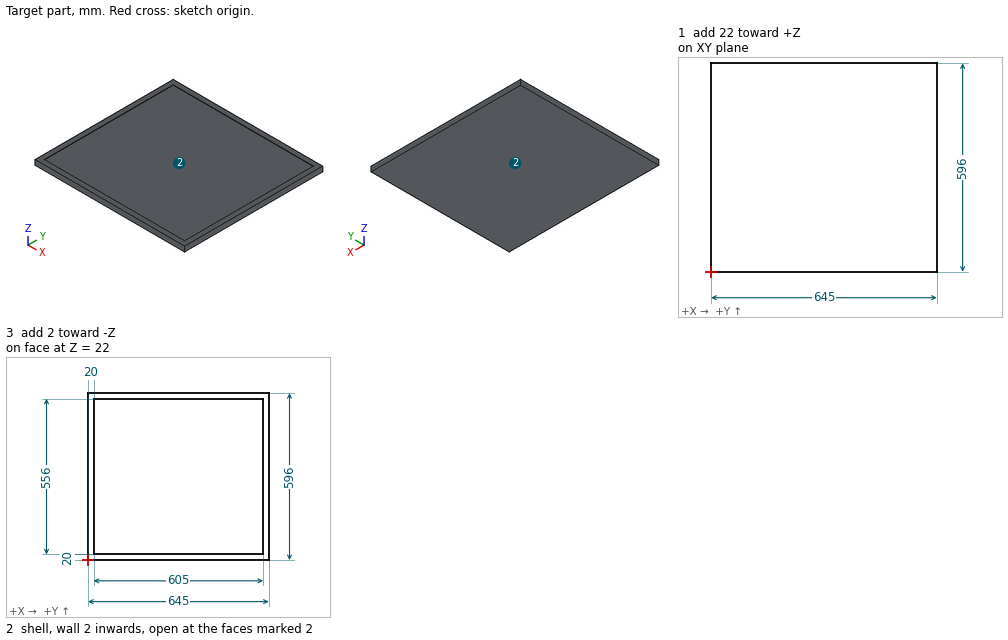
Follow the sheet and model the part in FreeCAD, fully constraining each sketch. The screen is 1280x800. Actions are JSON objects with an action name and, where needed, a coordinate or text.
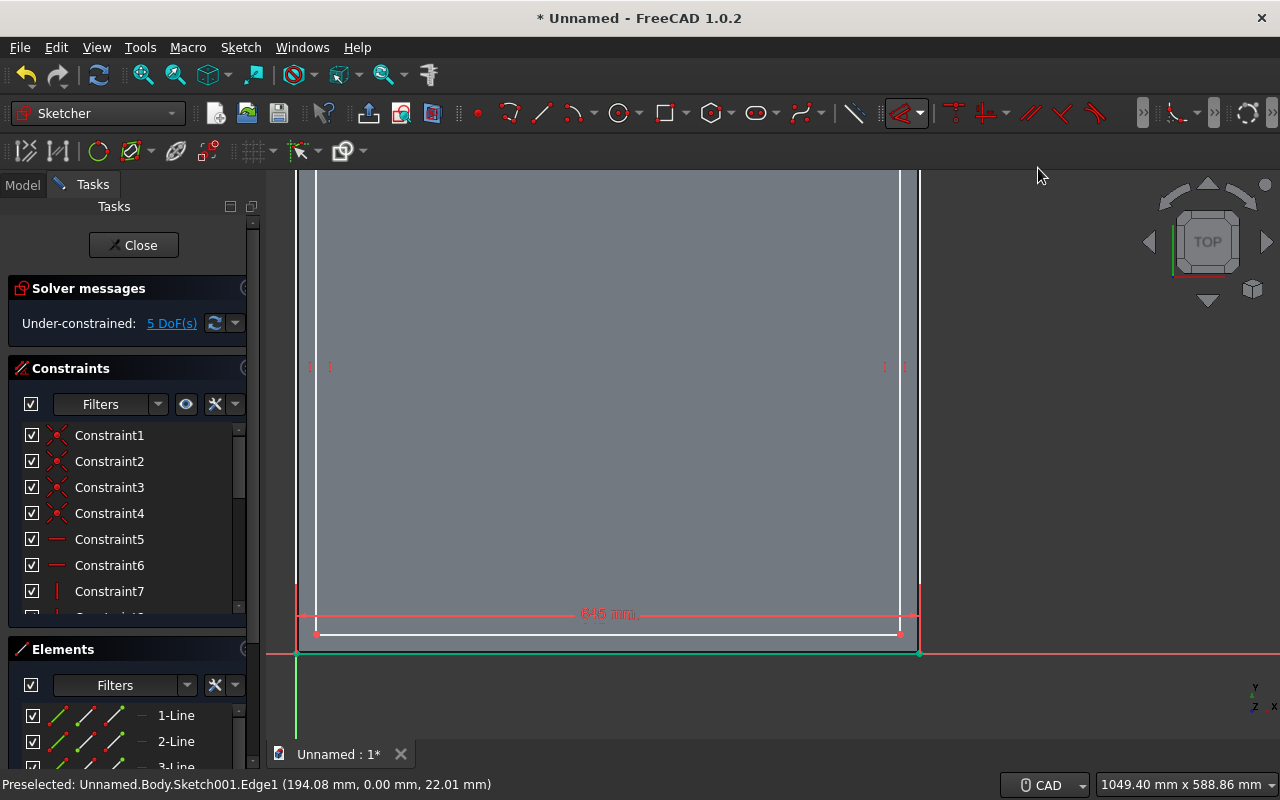
{"action": "left_click", "coordinate": [920, 481]}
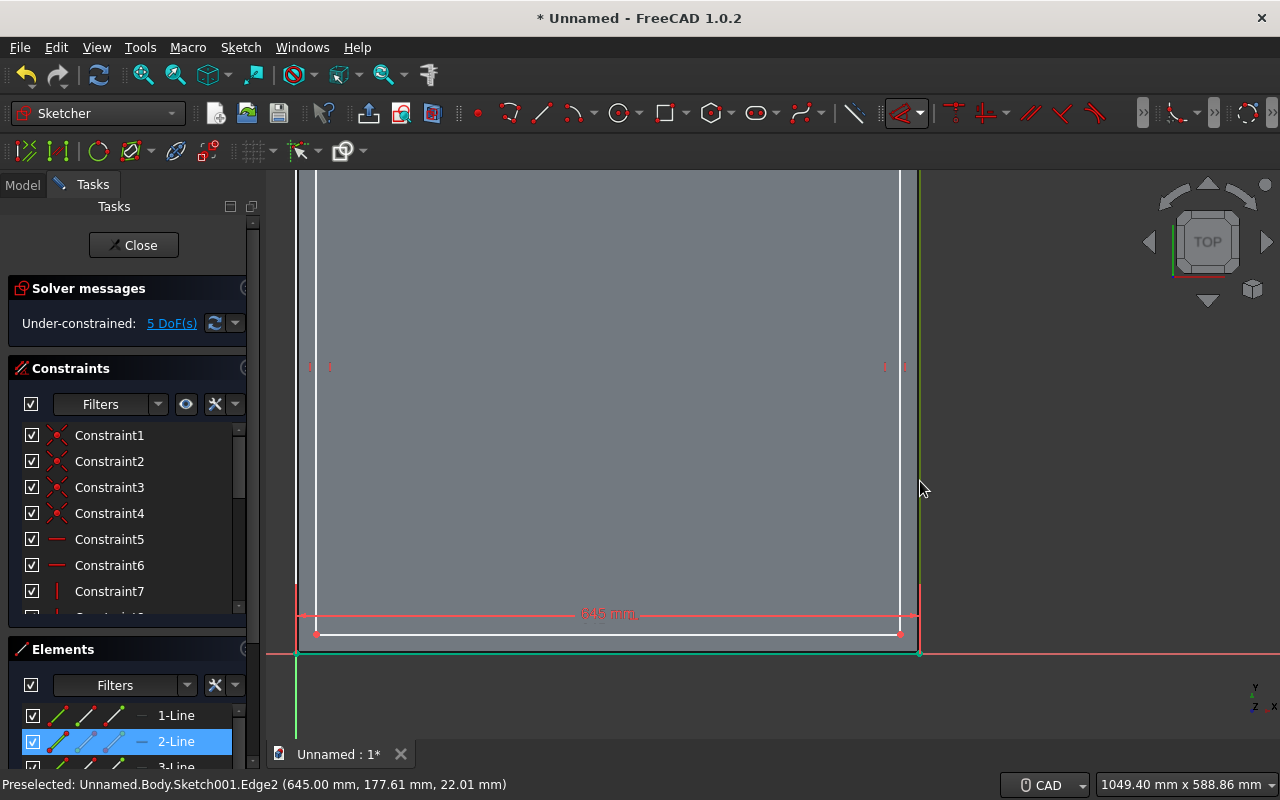
{"action": "key", "text": "i"}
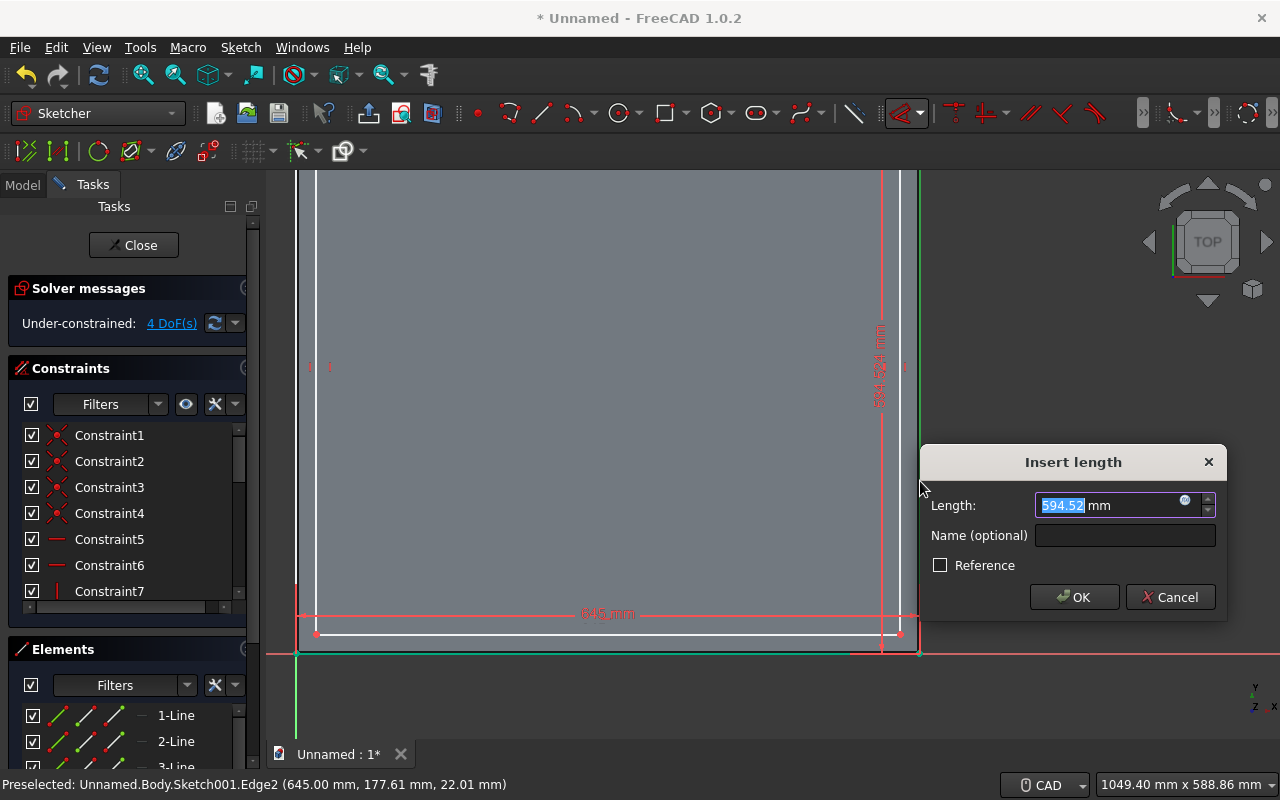
{"action": "type", "text": "596"}
{"action": "key", "text": "Return"}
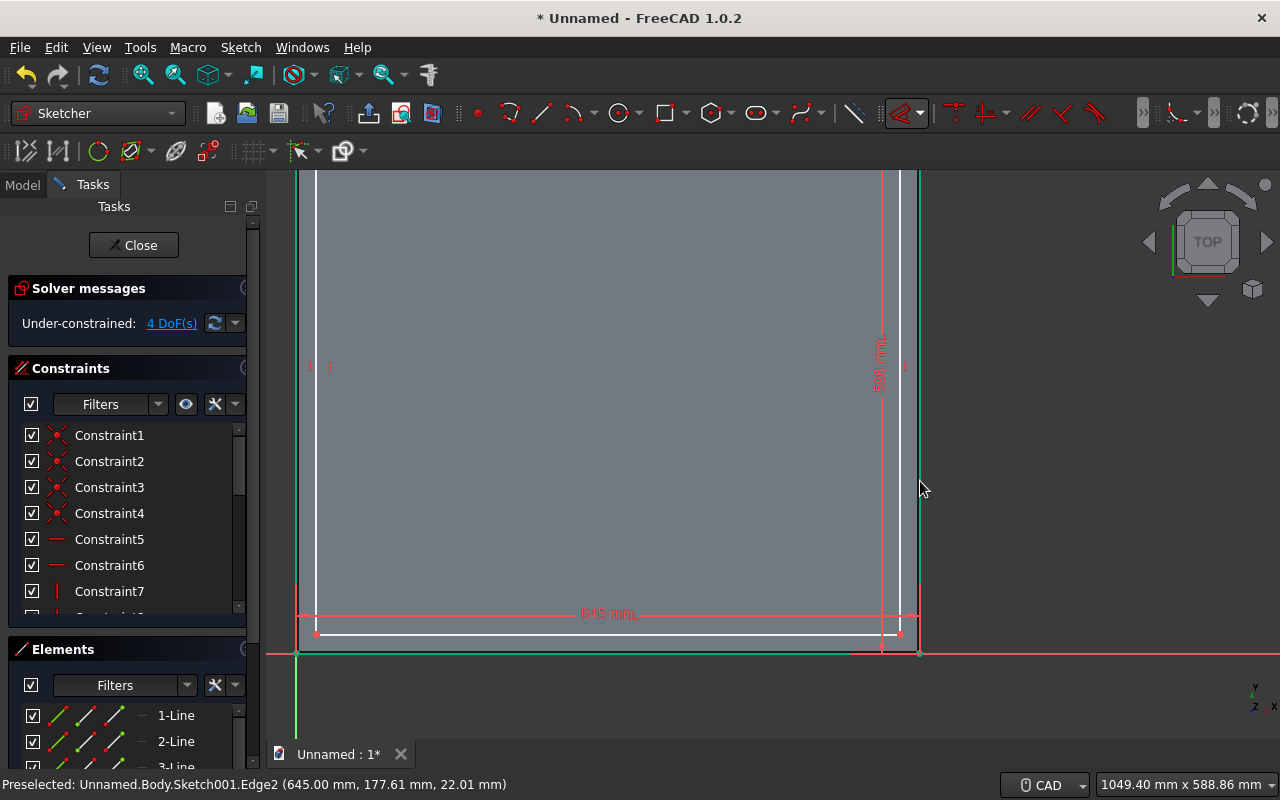
{"action": "left_click", "coordinate": [316, 259]}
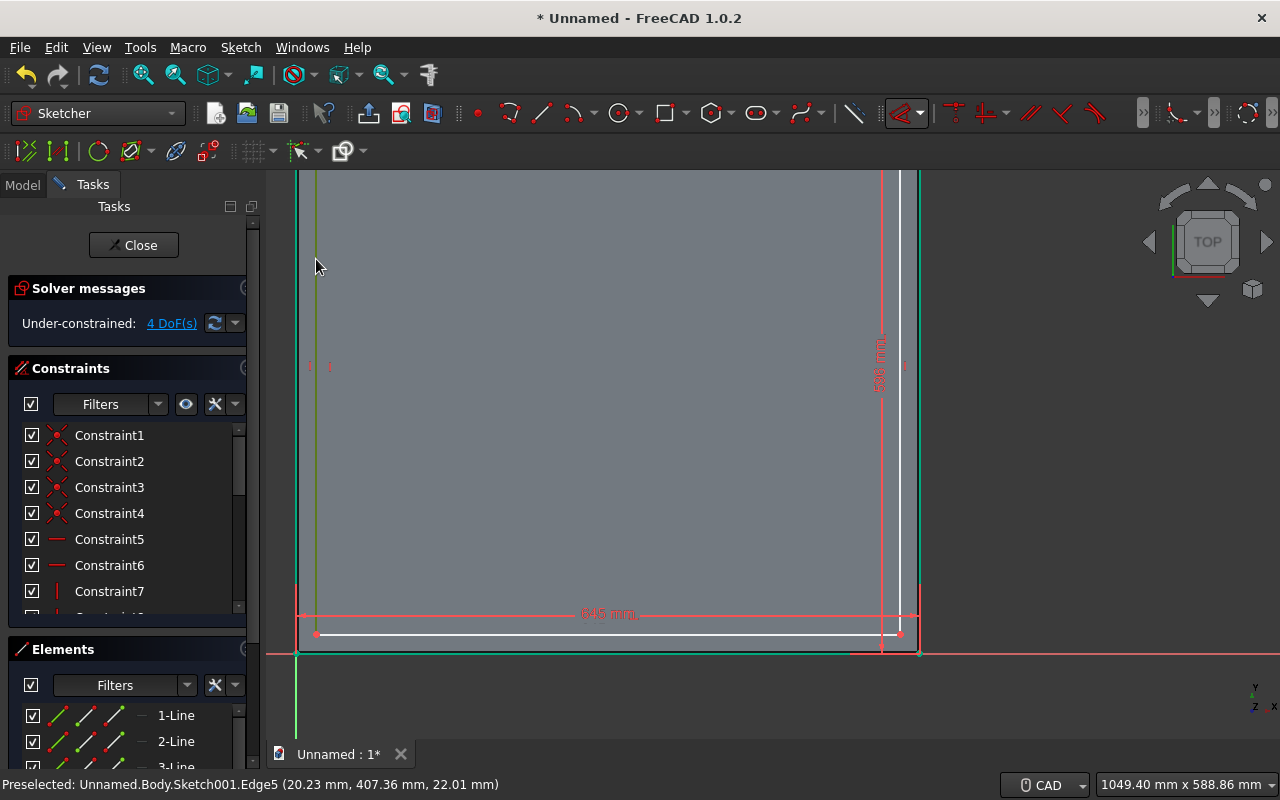
{"action": "key", "text": "i"}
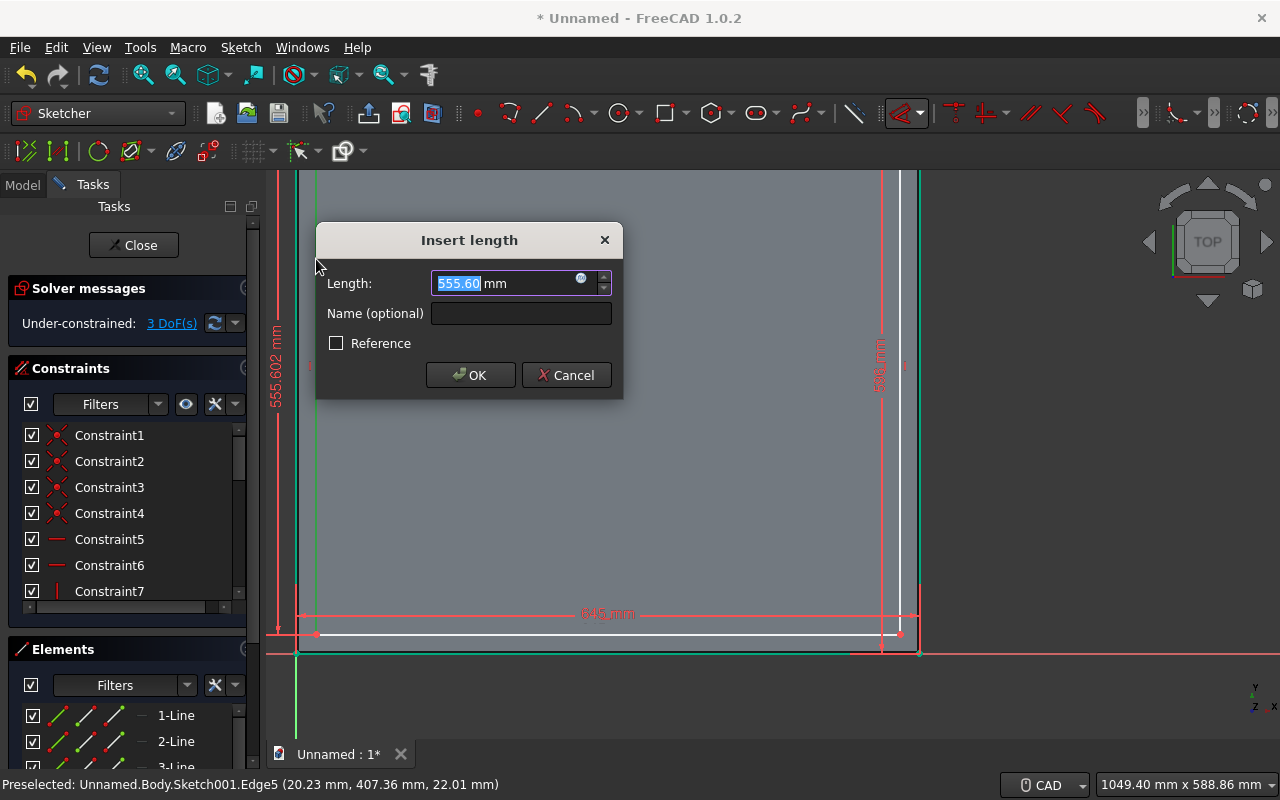
{"action": "type", "text": "556"}
{"action": "key", "text": "Return"}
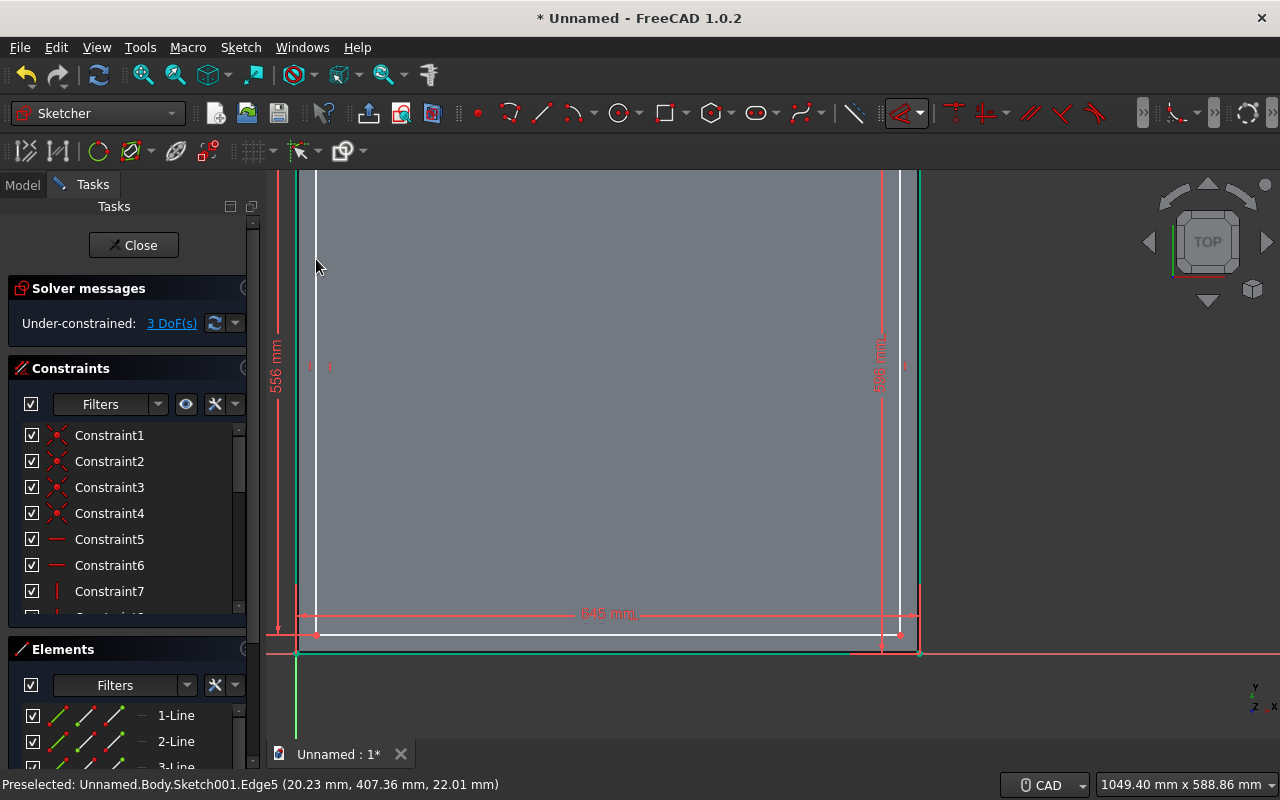
{"action": "left_click", "coordinate": [491, 635]}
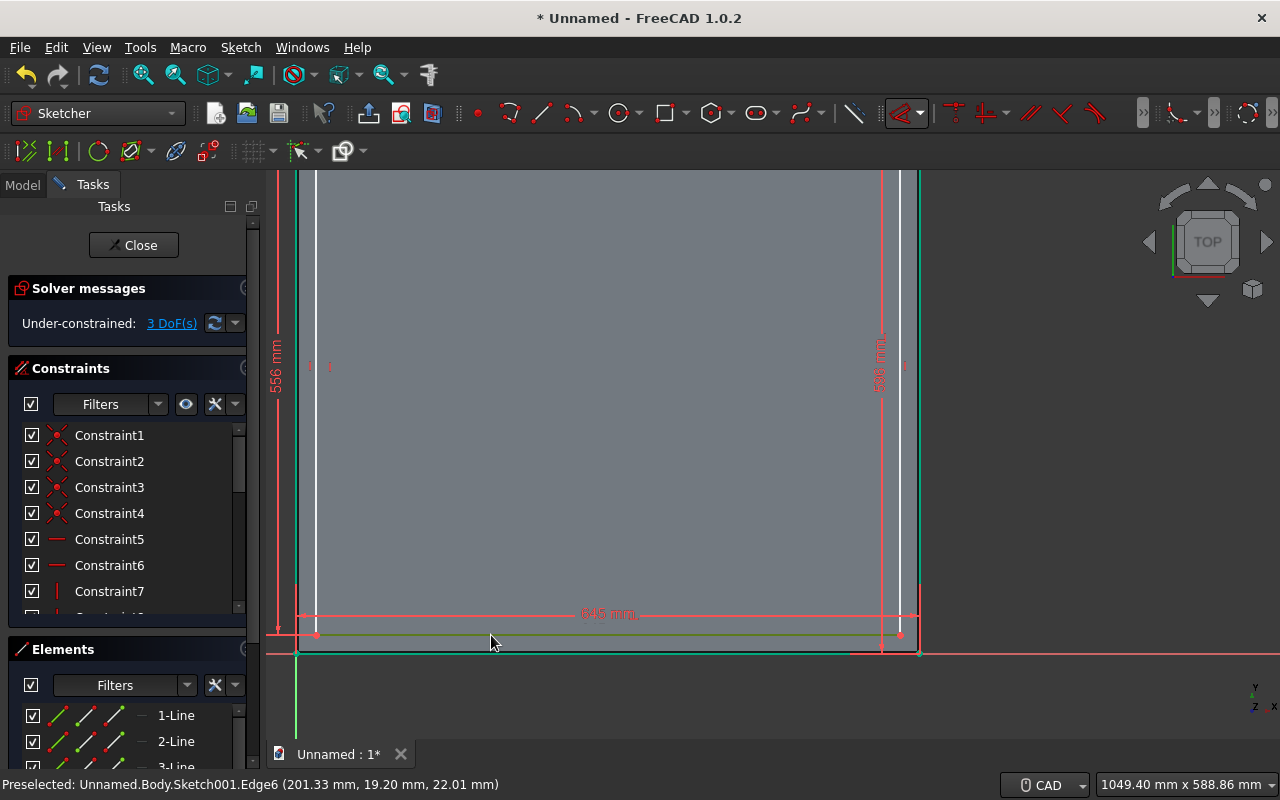
{"action": "left_click", "coordinate": [922, 114]}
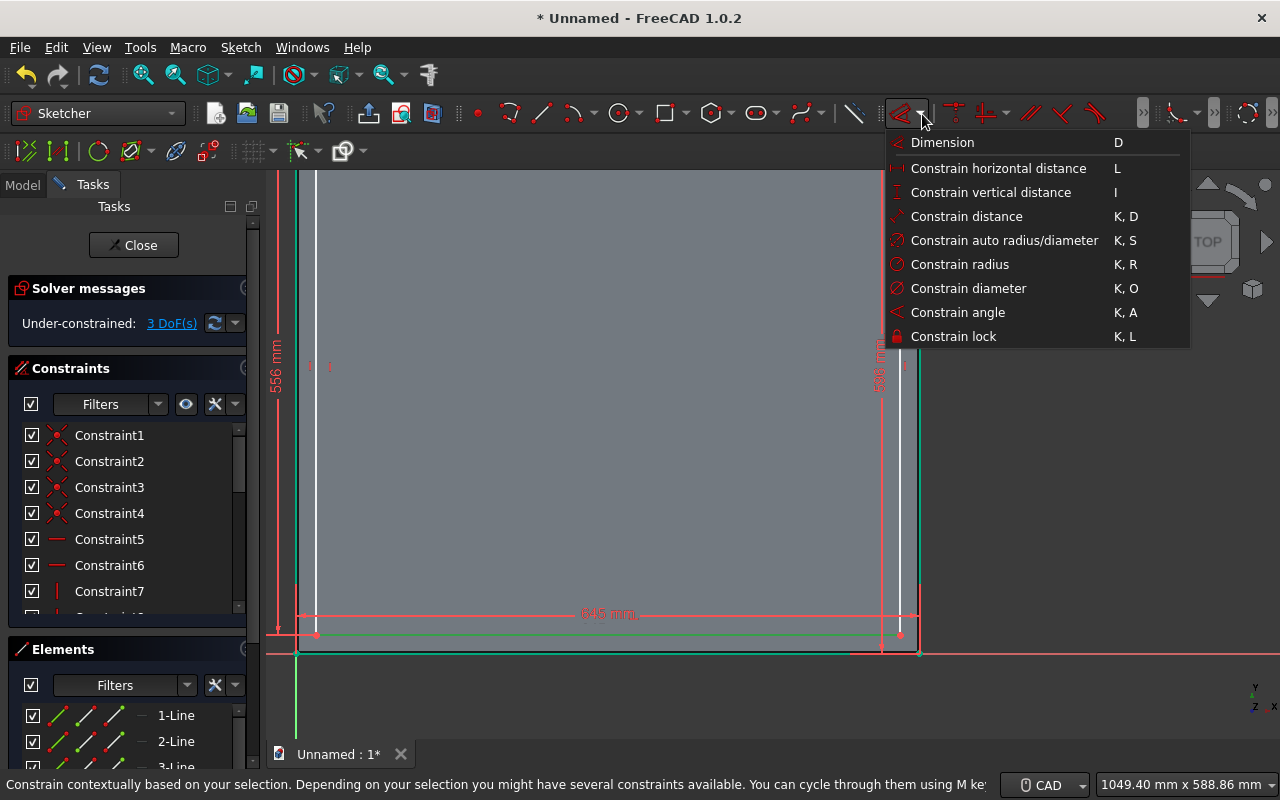
{"action": "left_click", "coordinate": [1038, 168]}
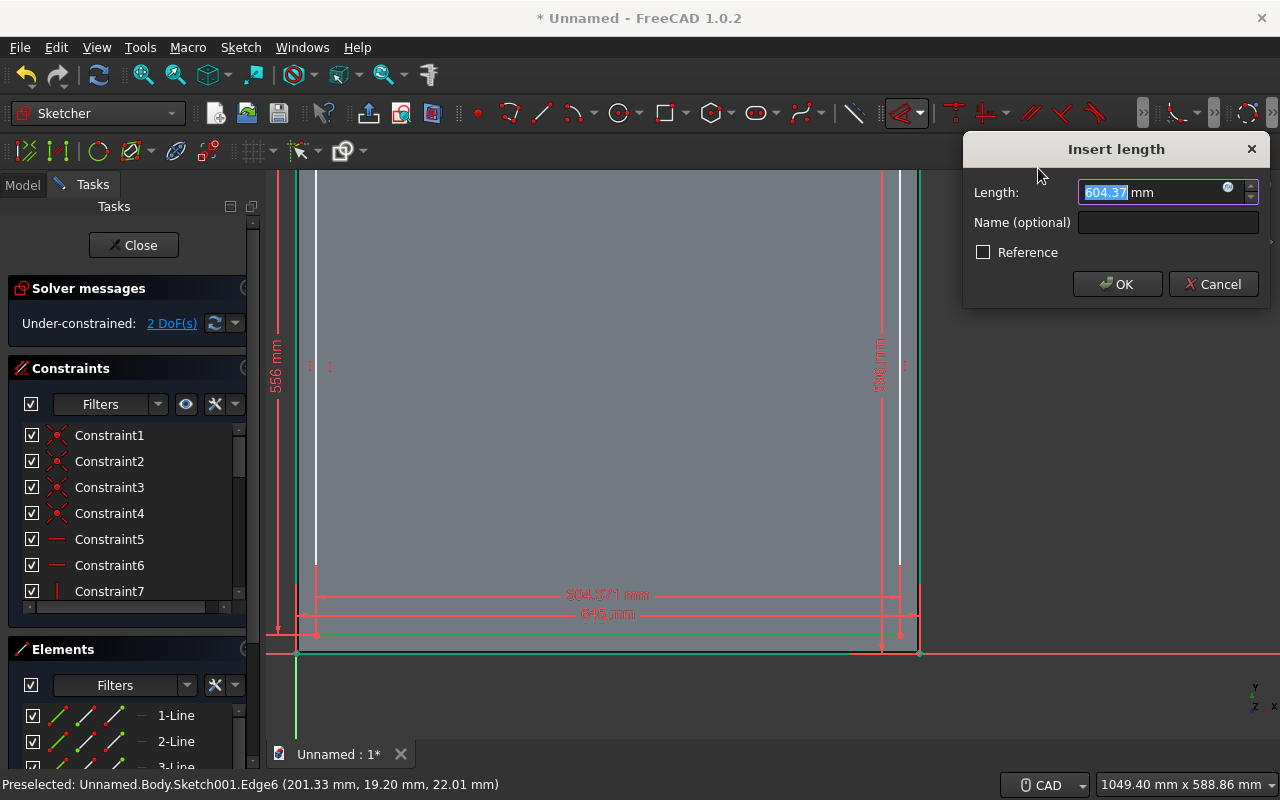
{"action": "type", "text": "605"}
{"action": "key", "text": "Return"}